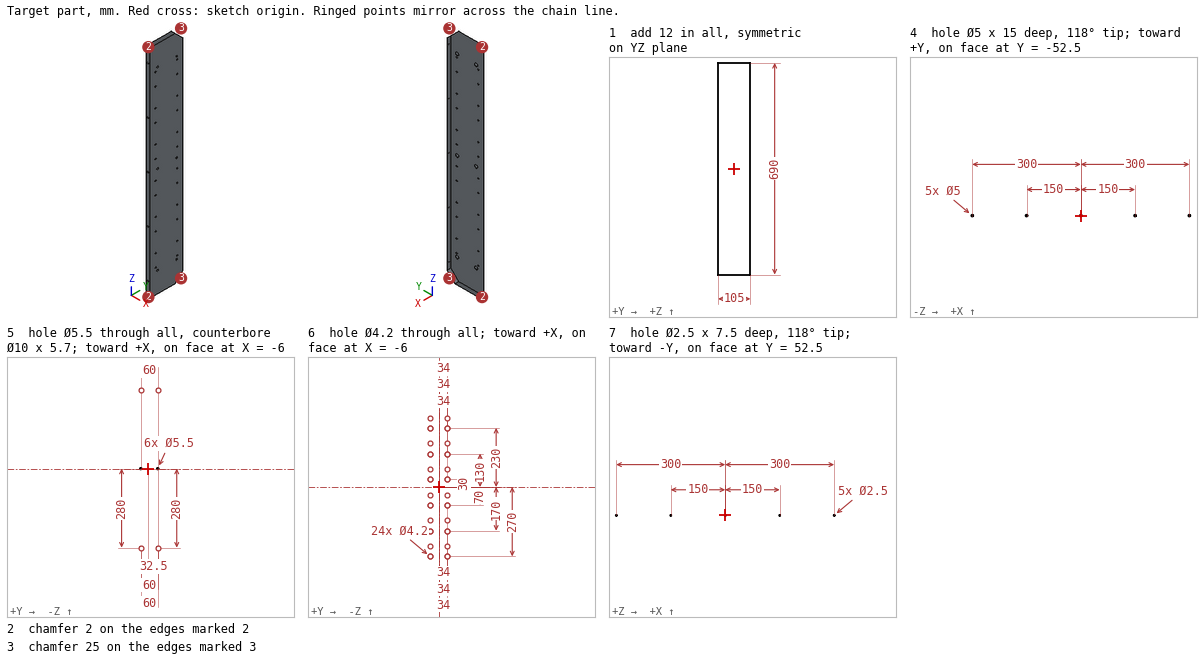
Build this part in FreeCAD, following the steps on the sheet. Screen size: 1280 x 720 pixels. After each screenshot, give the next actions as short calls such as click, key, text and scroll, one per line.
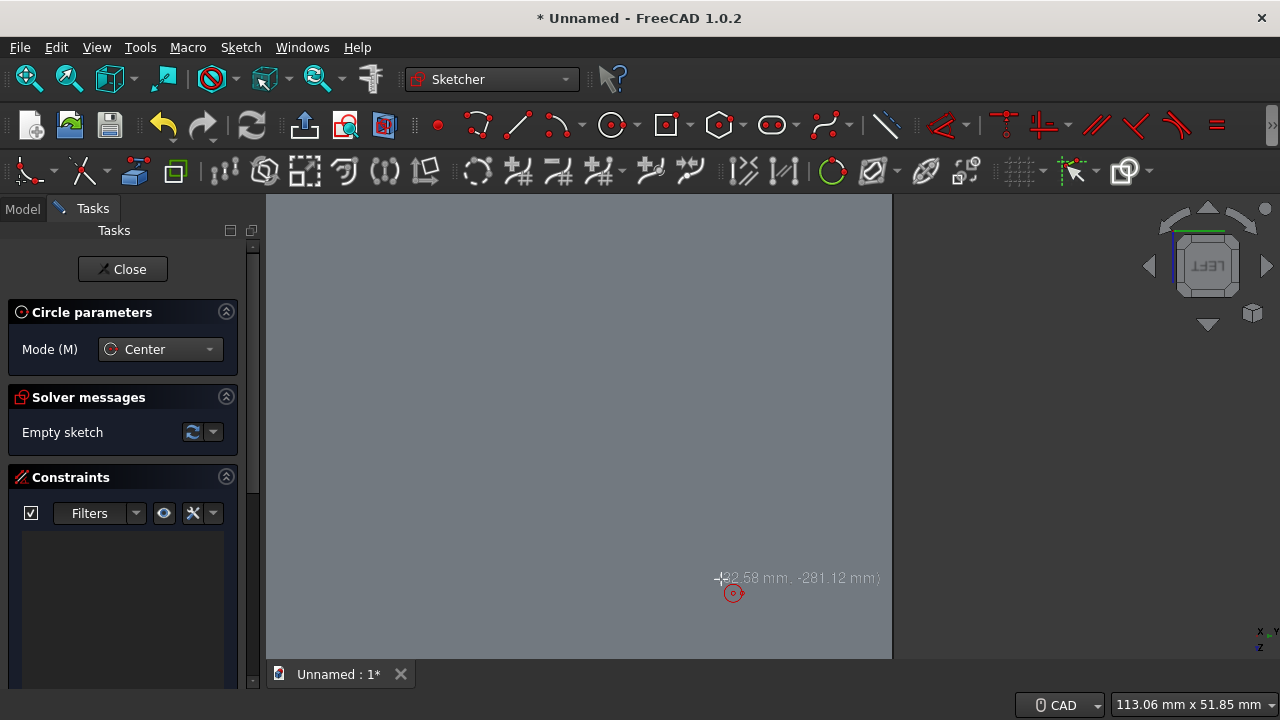
scroll(721, 580, down, 14)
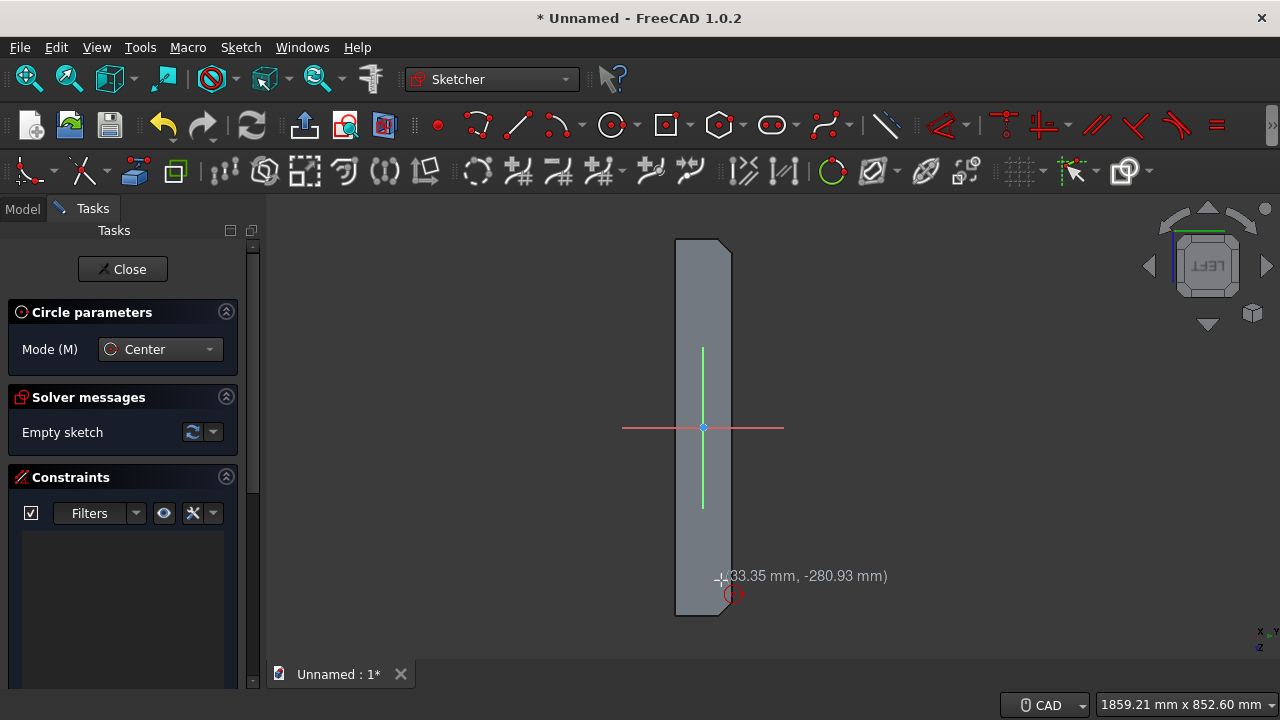
click(721, 580)
move(722, 579)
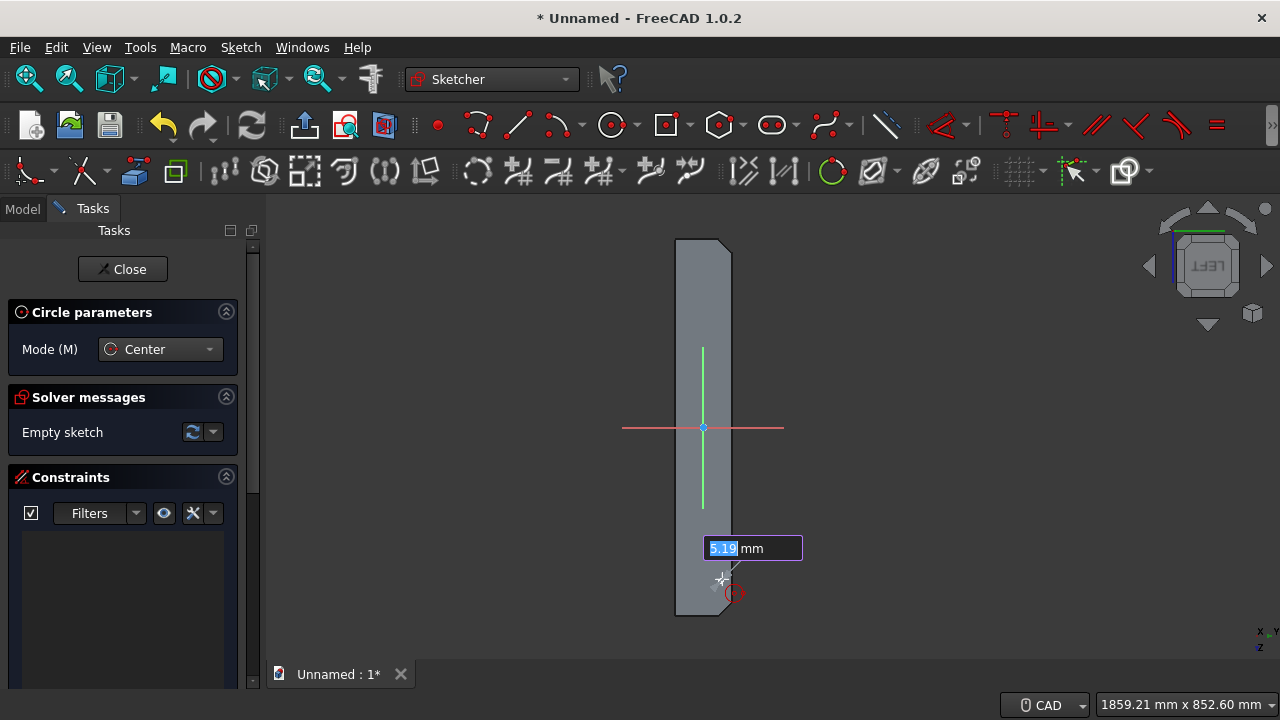
text(5.5)
key(Return)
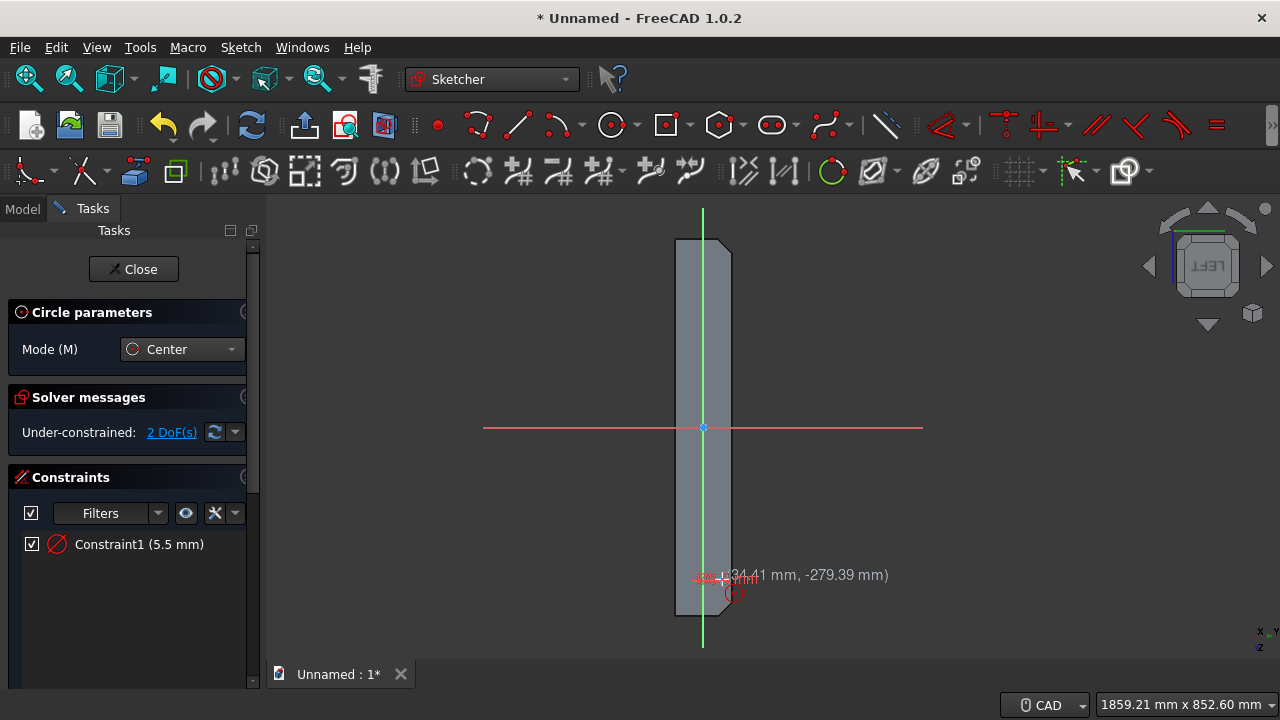
scroll(688, 580, up, 14)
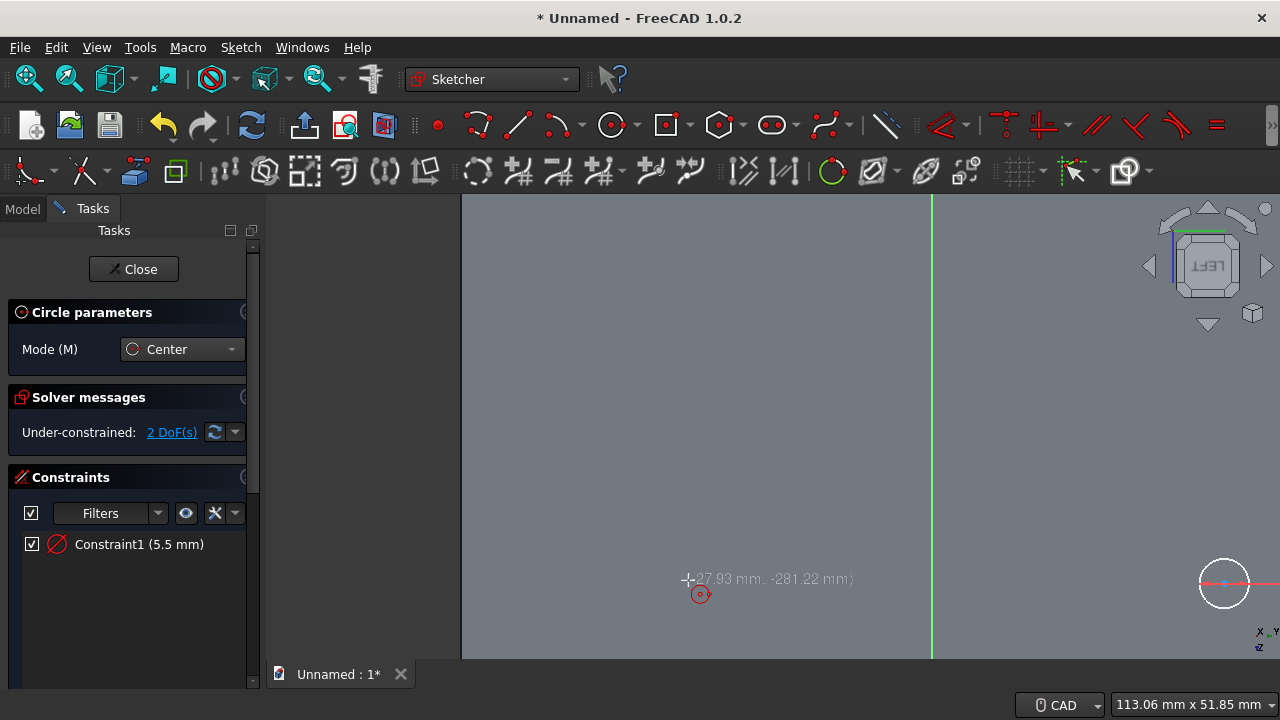
scroll(688, 580, down, 14)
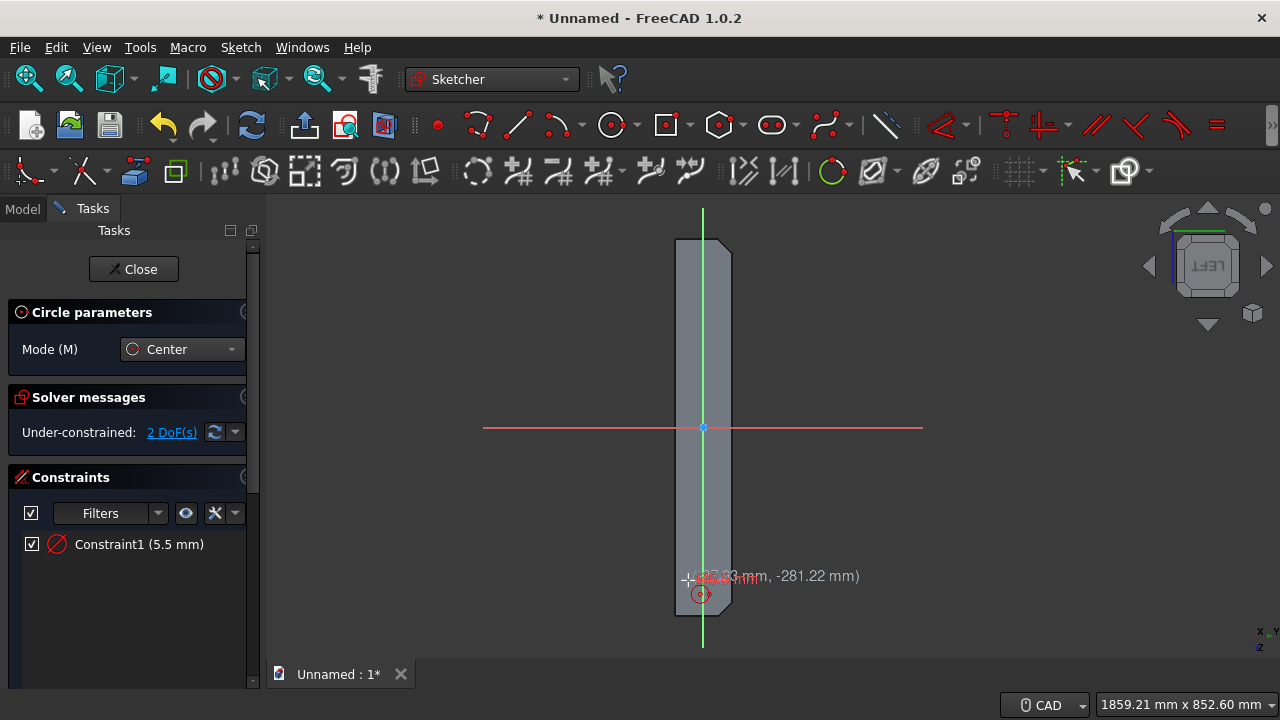
click(688, 580)
move(687, 579)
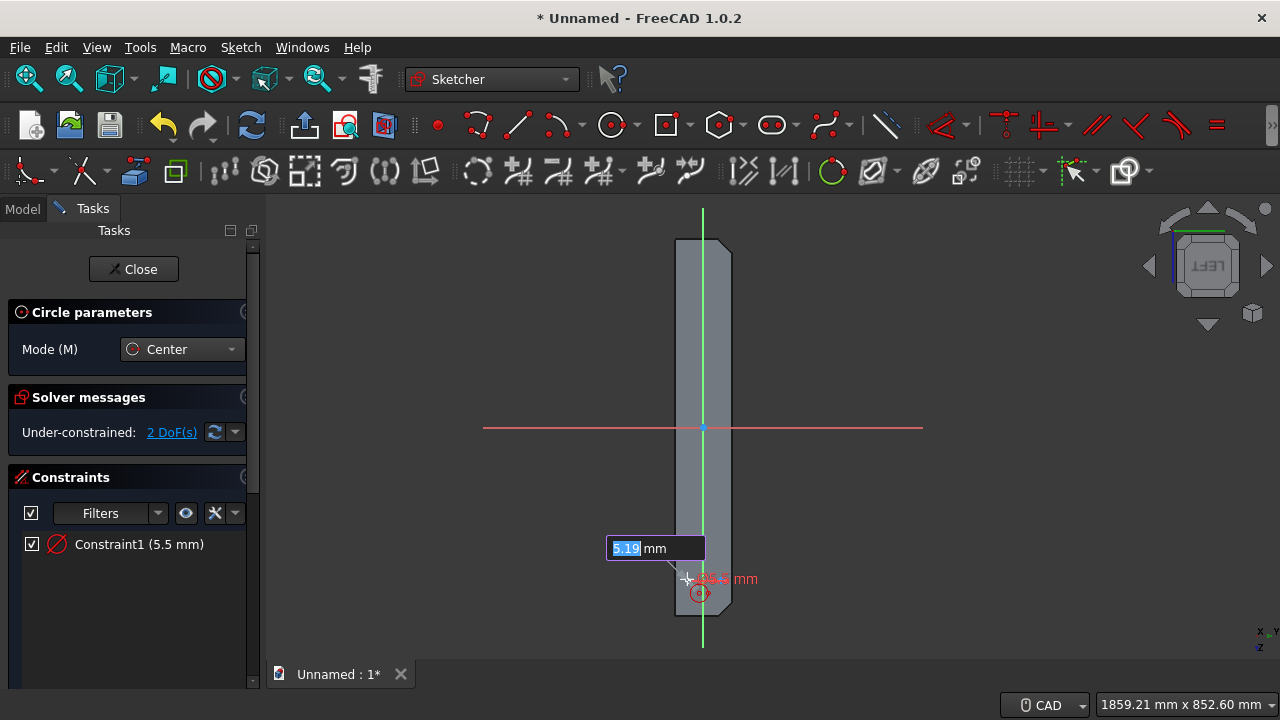
text(5.5)
key(Return)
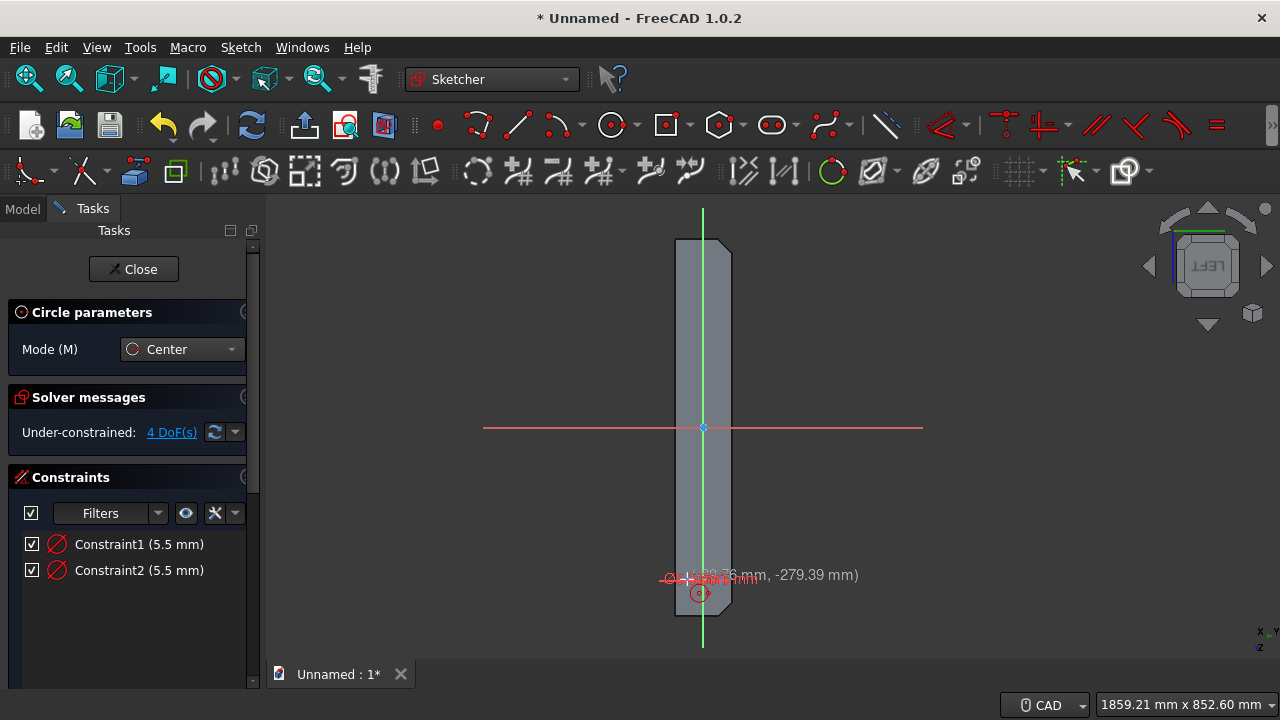
scroll(721, 428, up, 14)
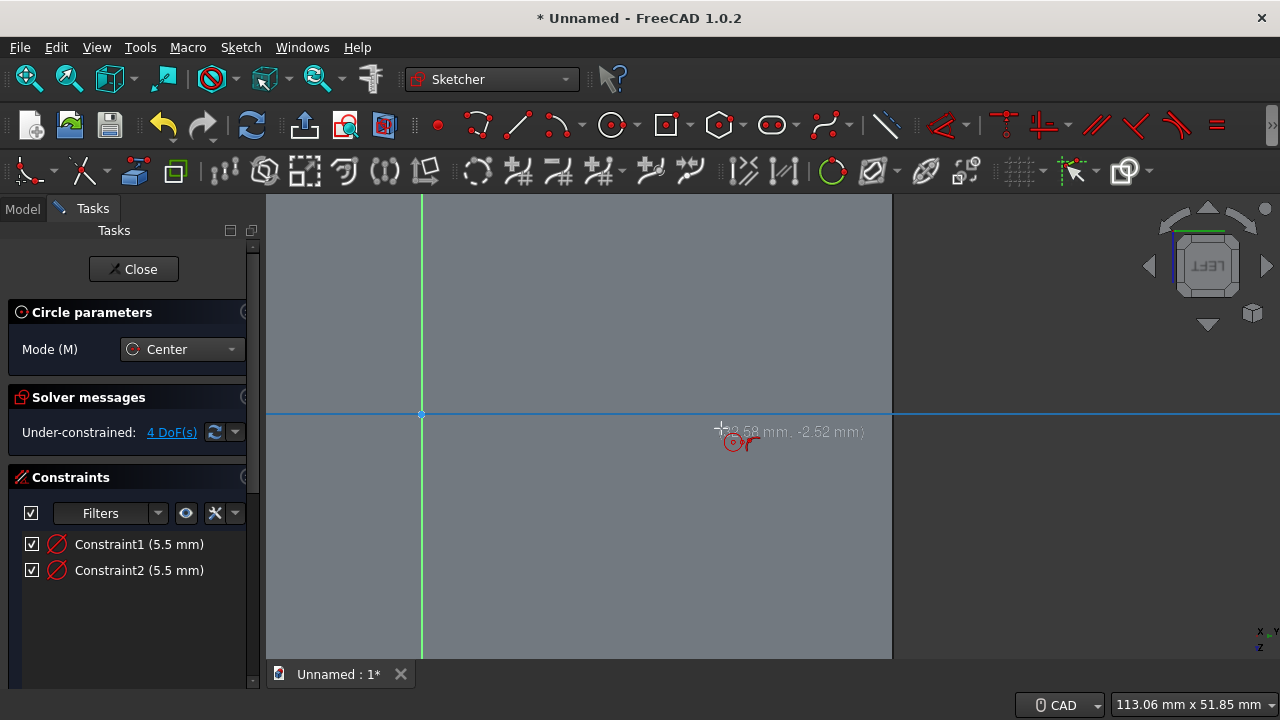
scroll(721, 427, down, 14)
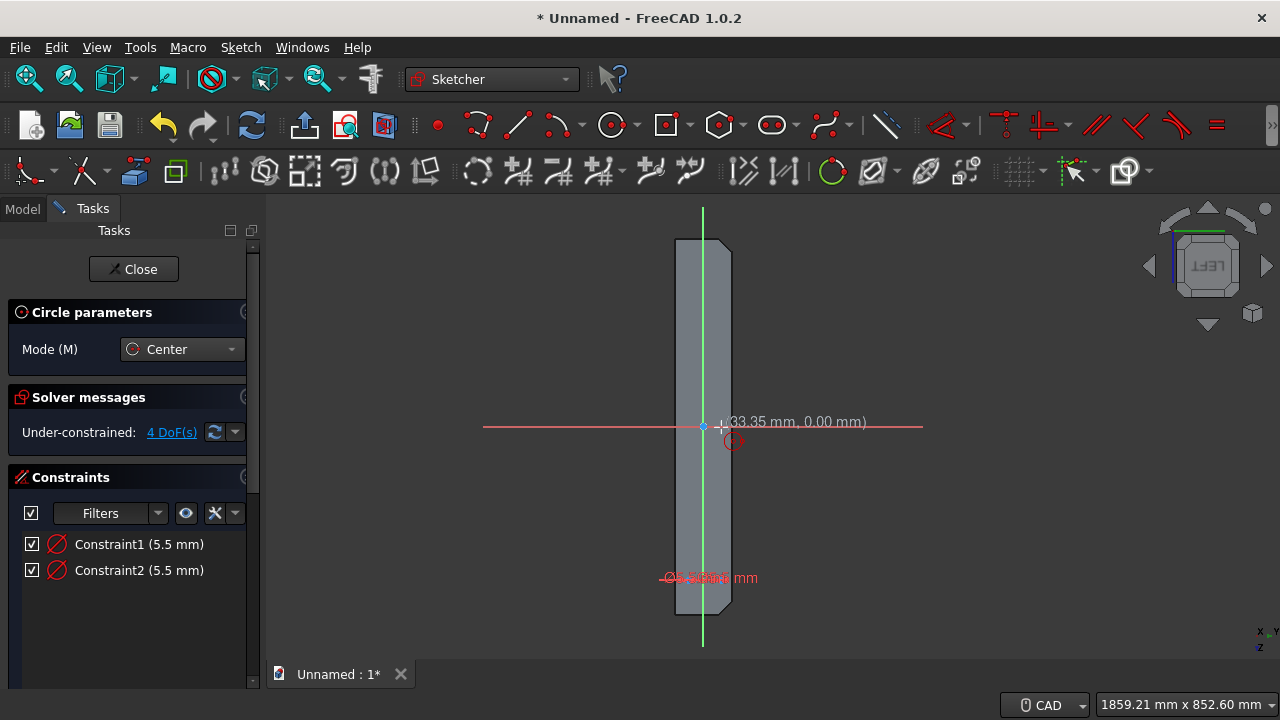
click(721, 427)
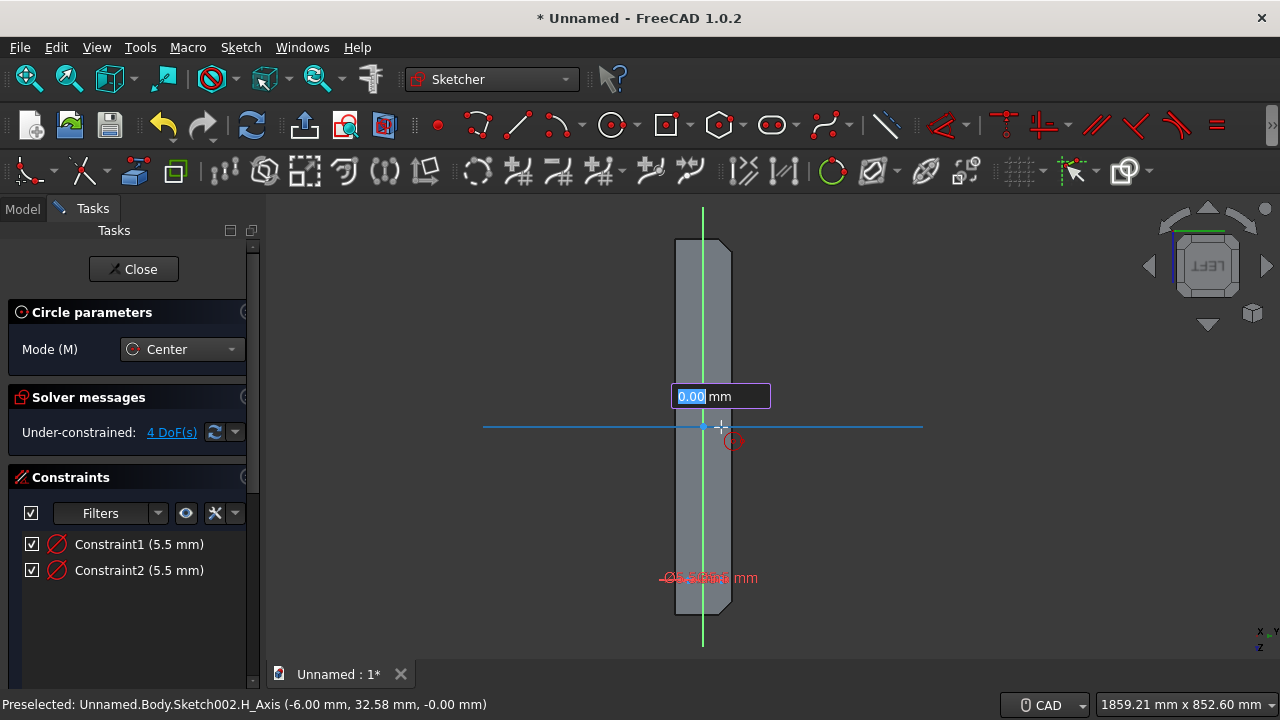
scroll(721, 425, up, 13)
move(722, 422)